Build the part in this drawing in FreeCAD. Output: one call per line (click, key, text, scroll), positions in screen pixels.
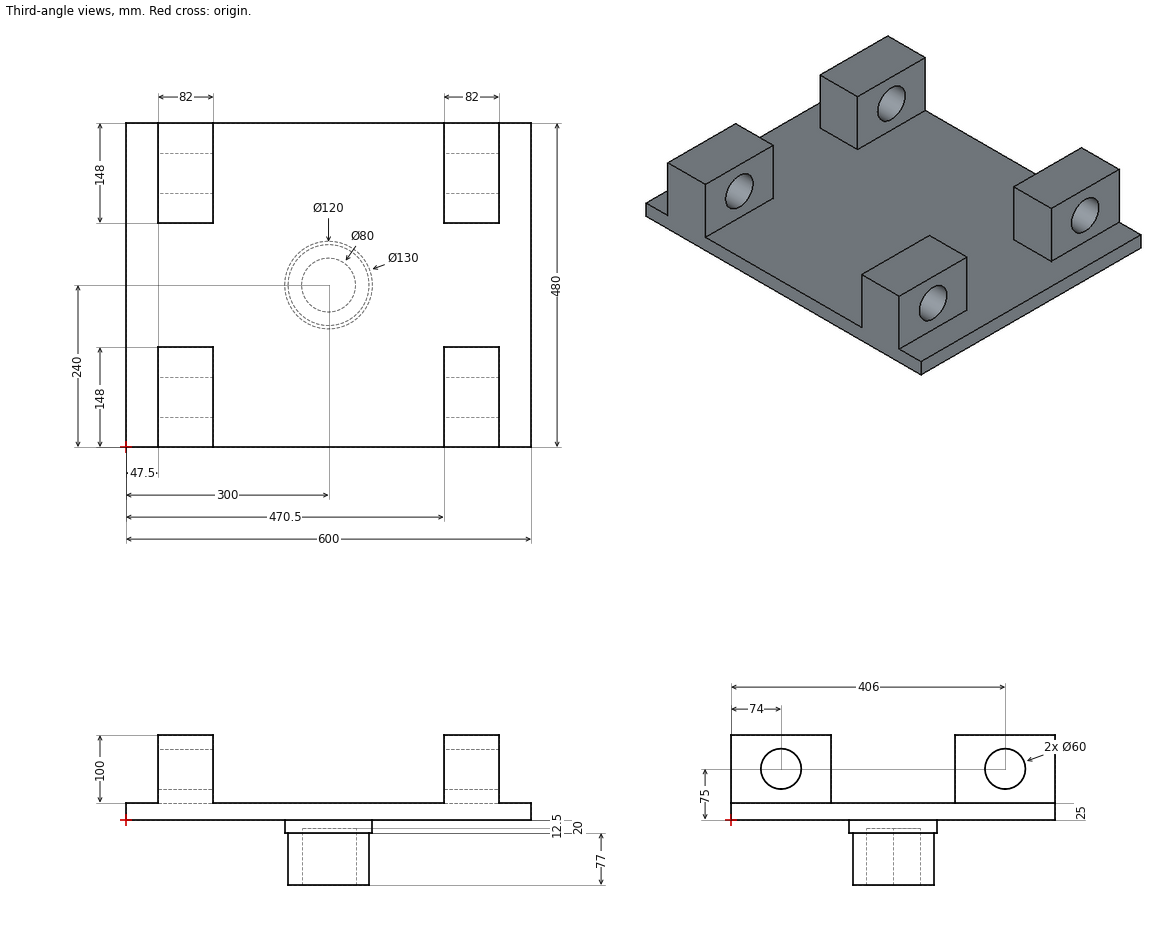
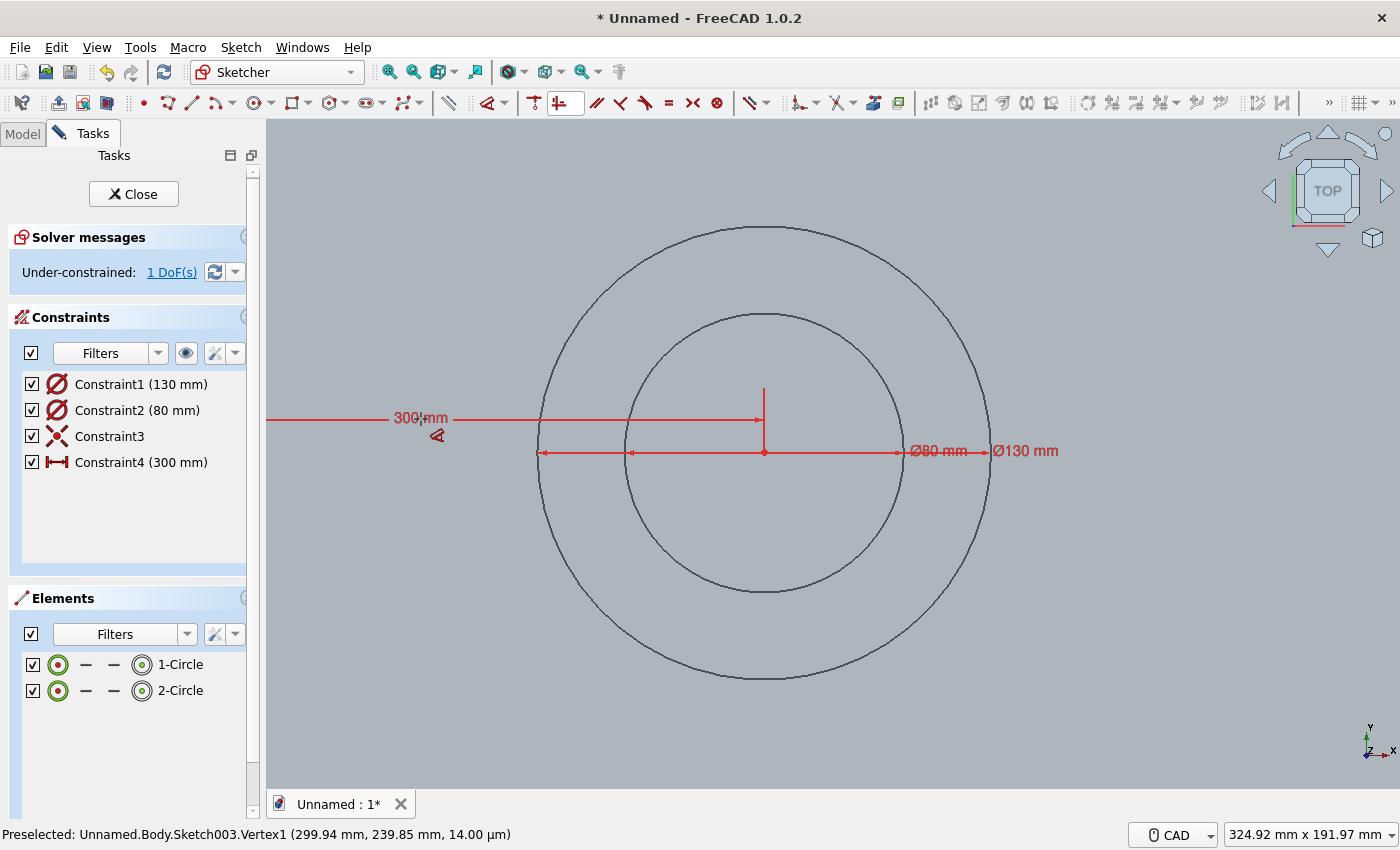
click(764, 453)
click(798, 607)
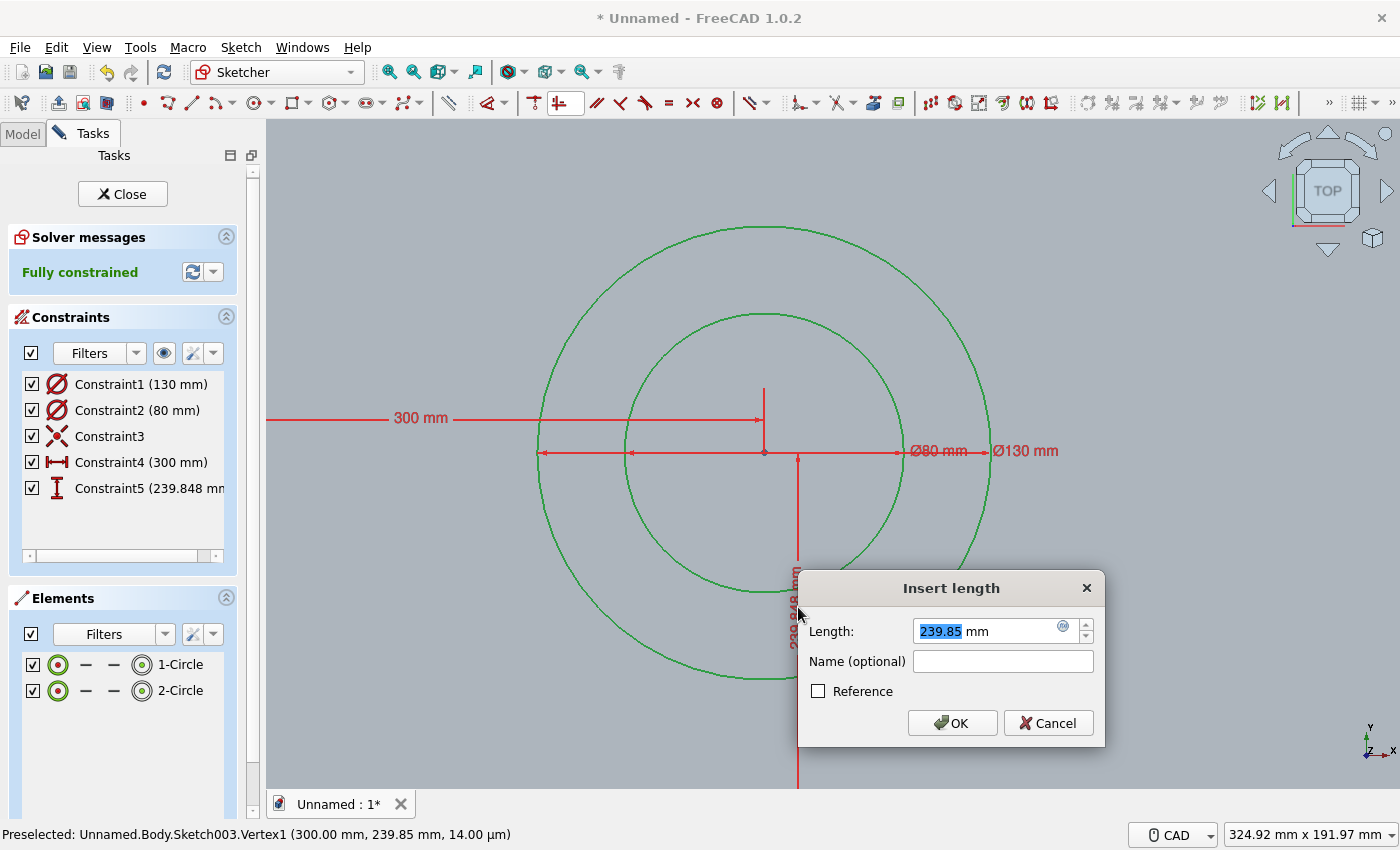
text(240)
key(Return)
key(Escape)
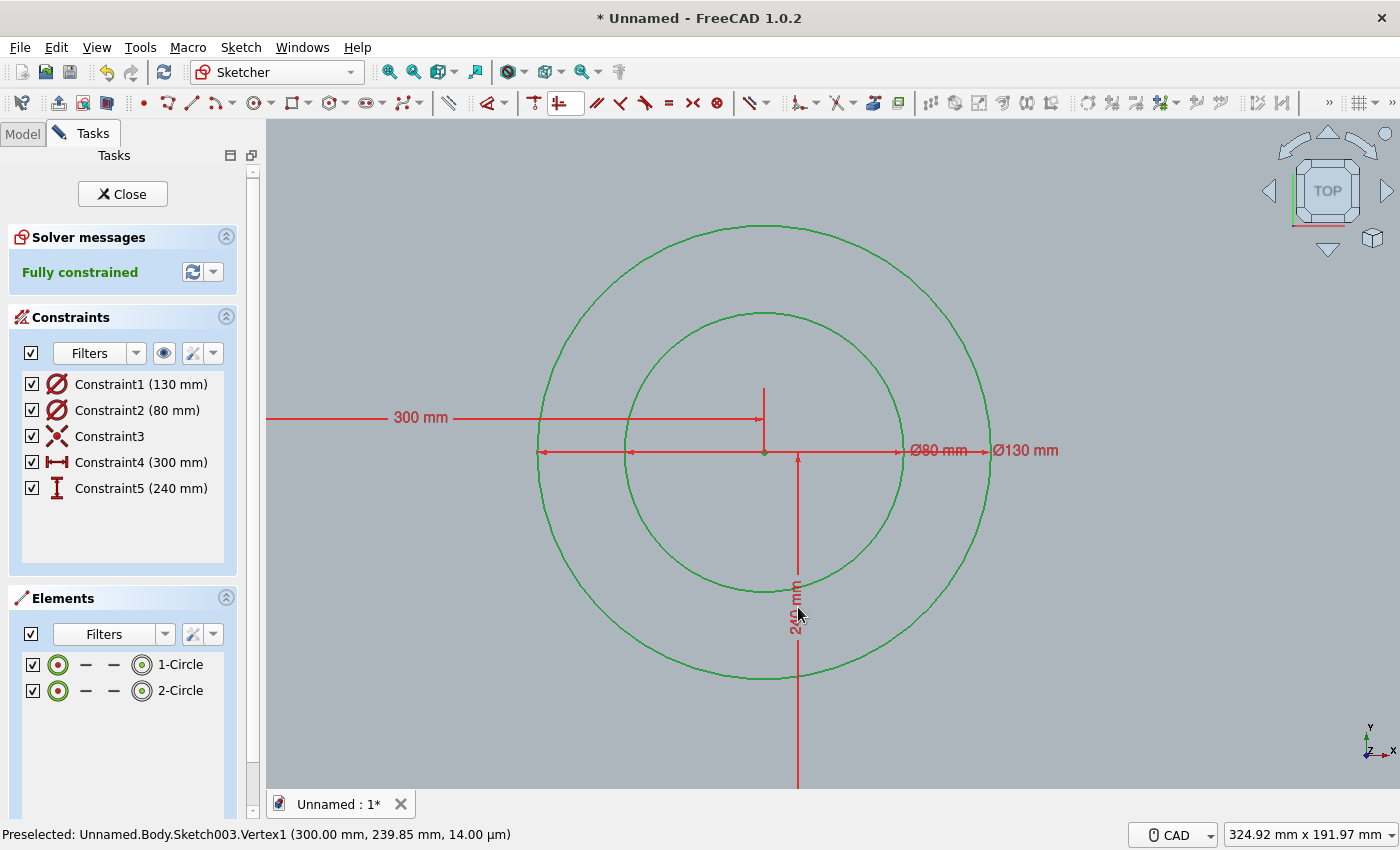
click(123, 194)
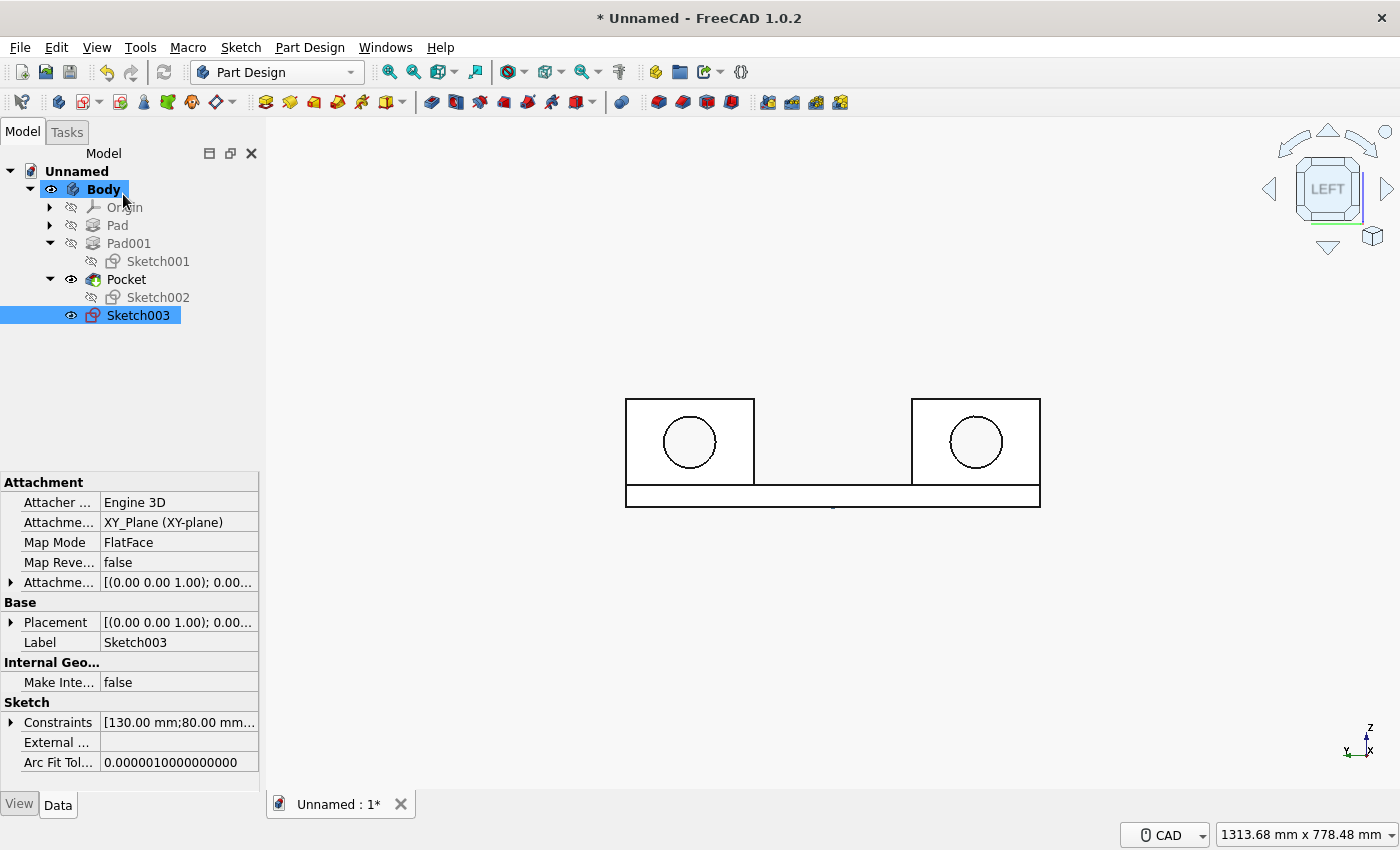
click(266, 102)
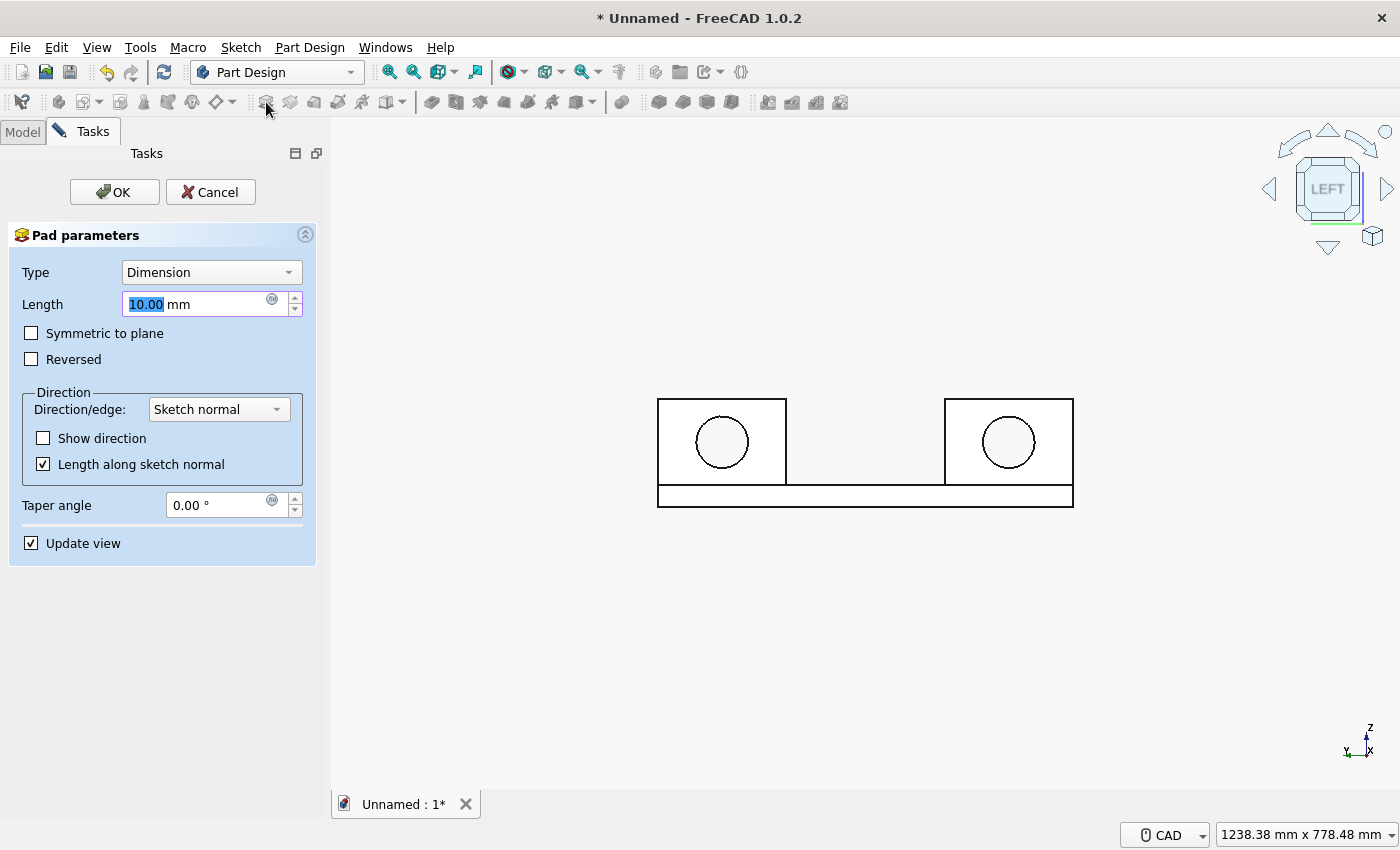
text(20)
key(Tab)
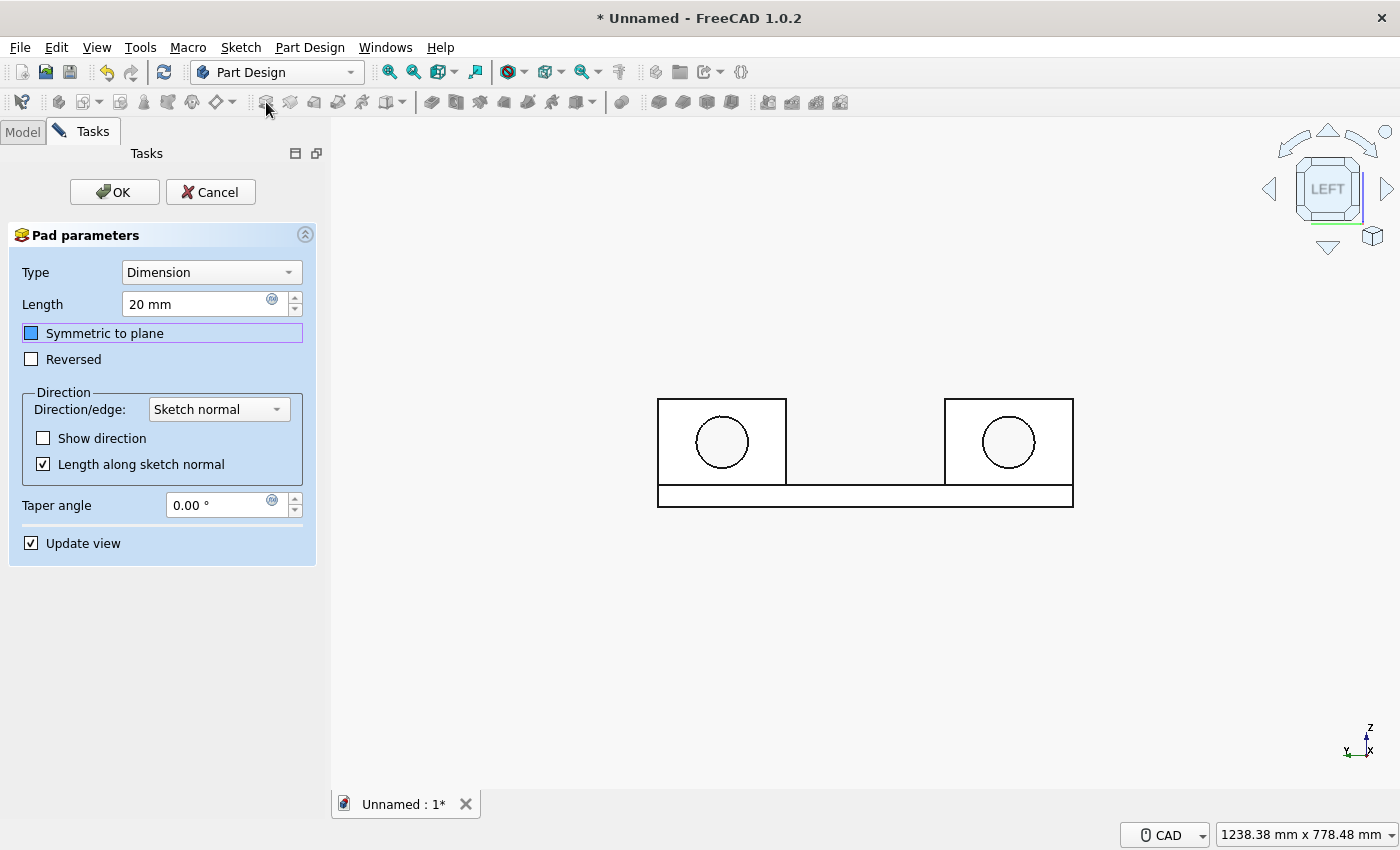
click(30, 359)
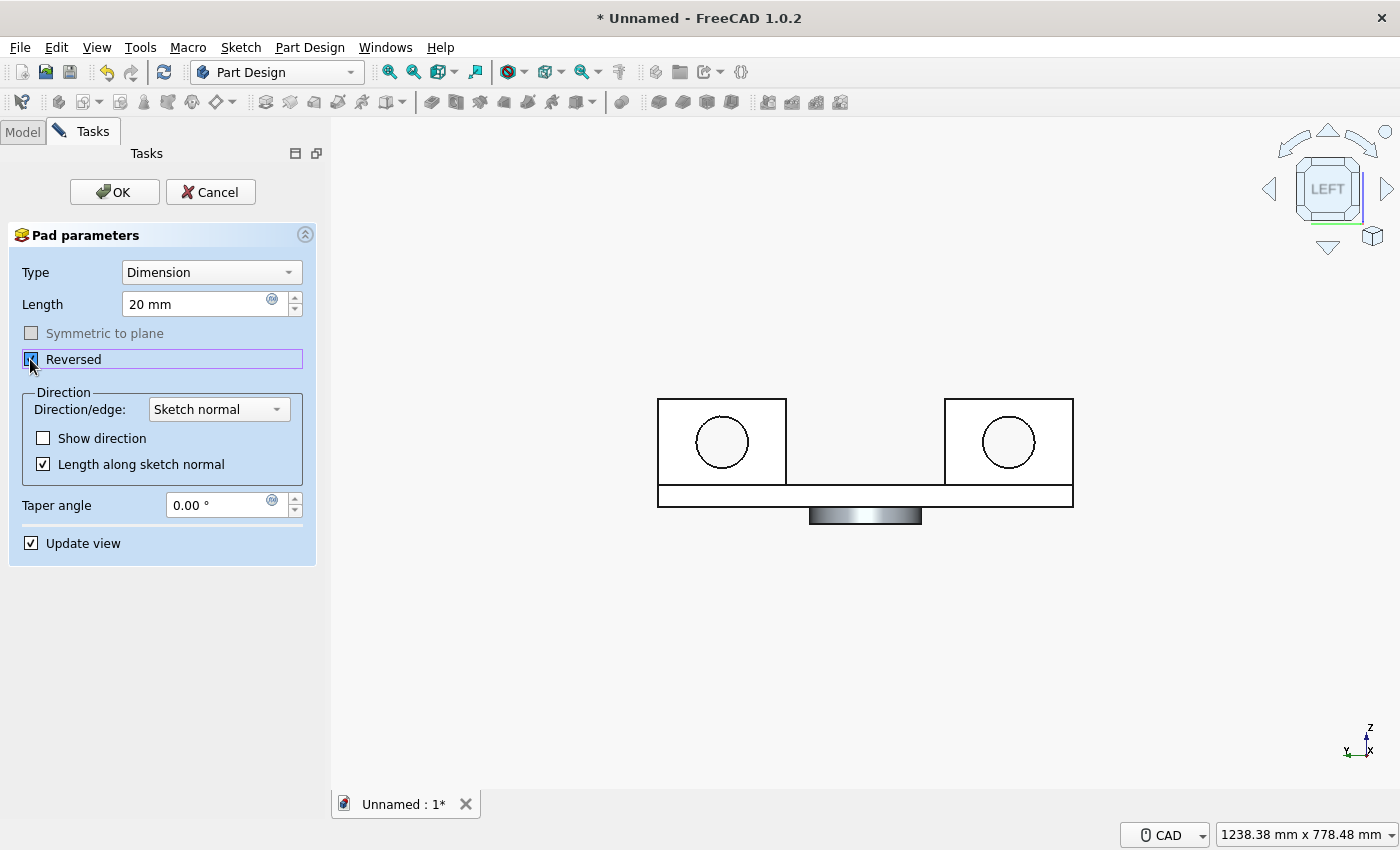
click(115, 192)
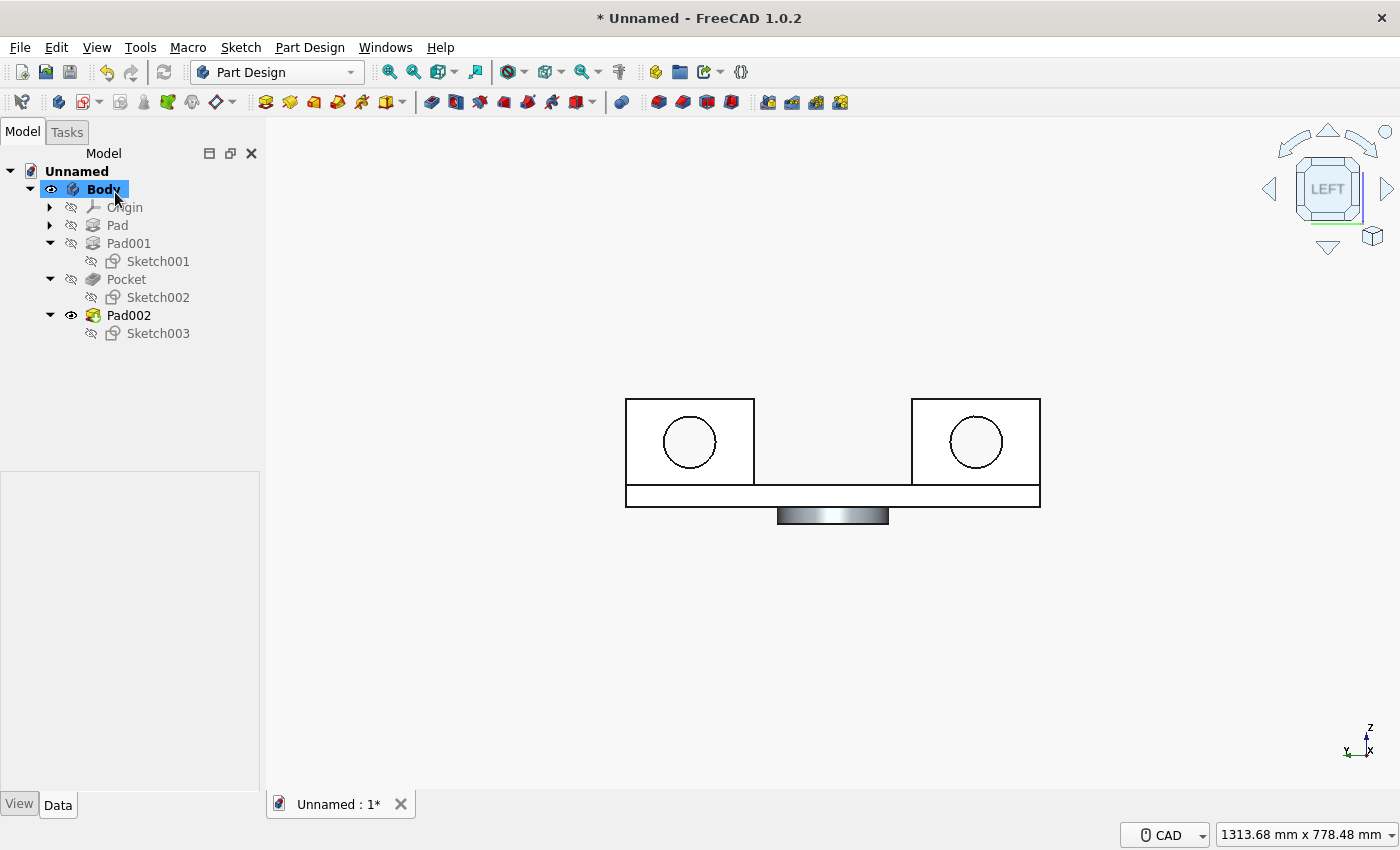
click(390, 72)